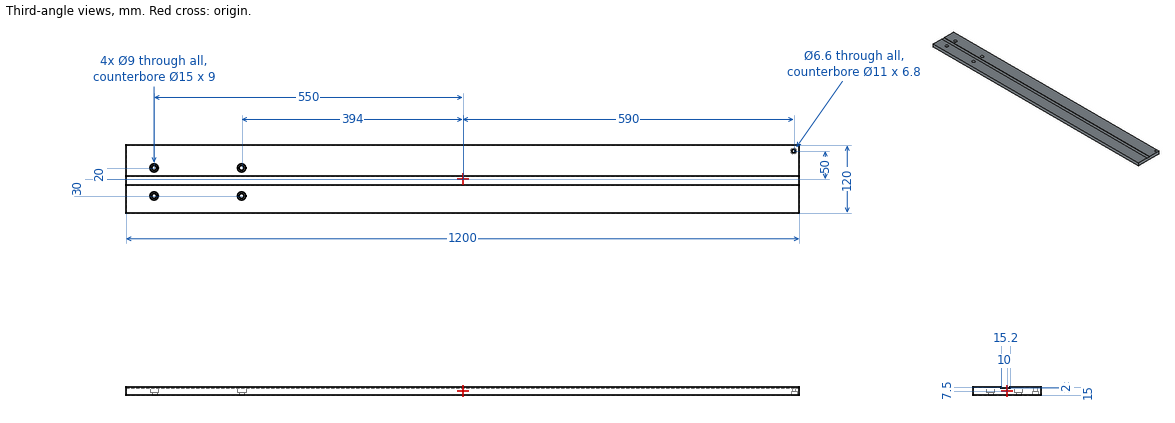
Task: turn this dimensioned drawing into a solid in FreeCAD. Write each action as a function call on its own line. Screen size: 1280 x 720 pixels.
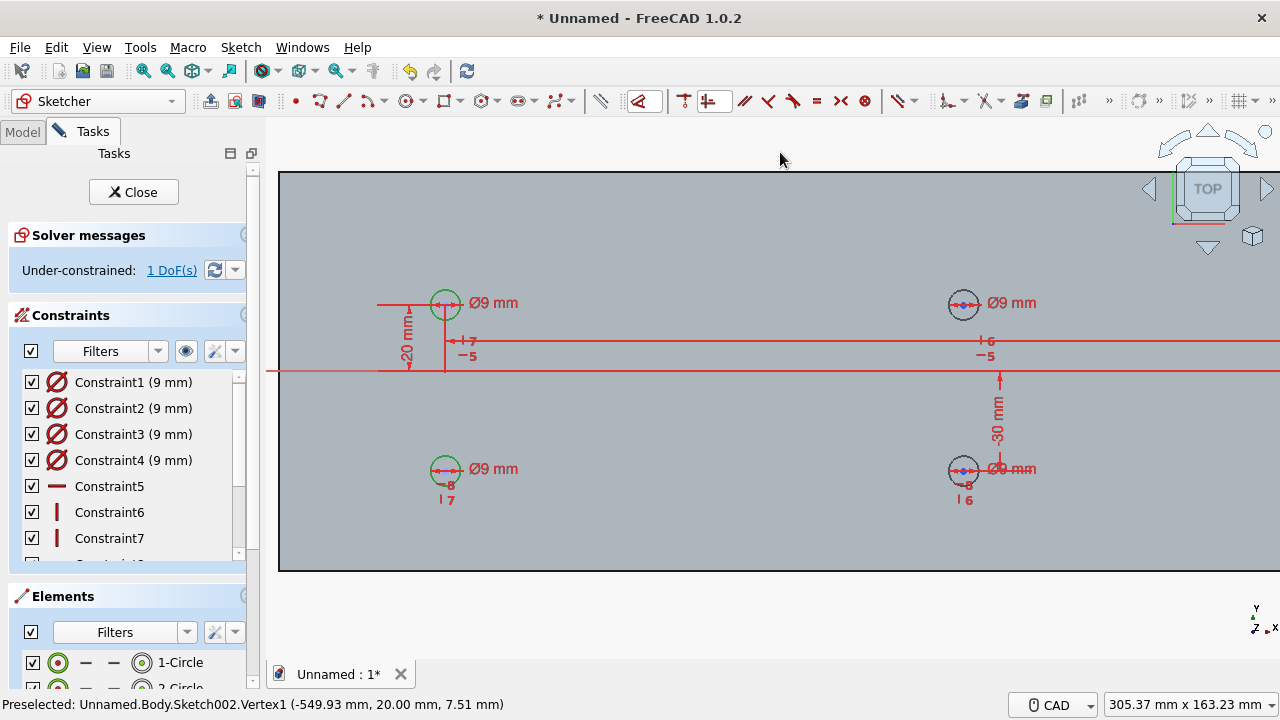
click(964, 305)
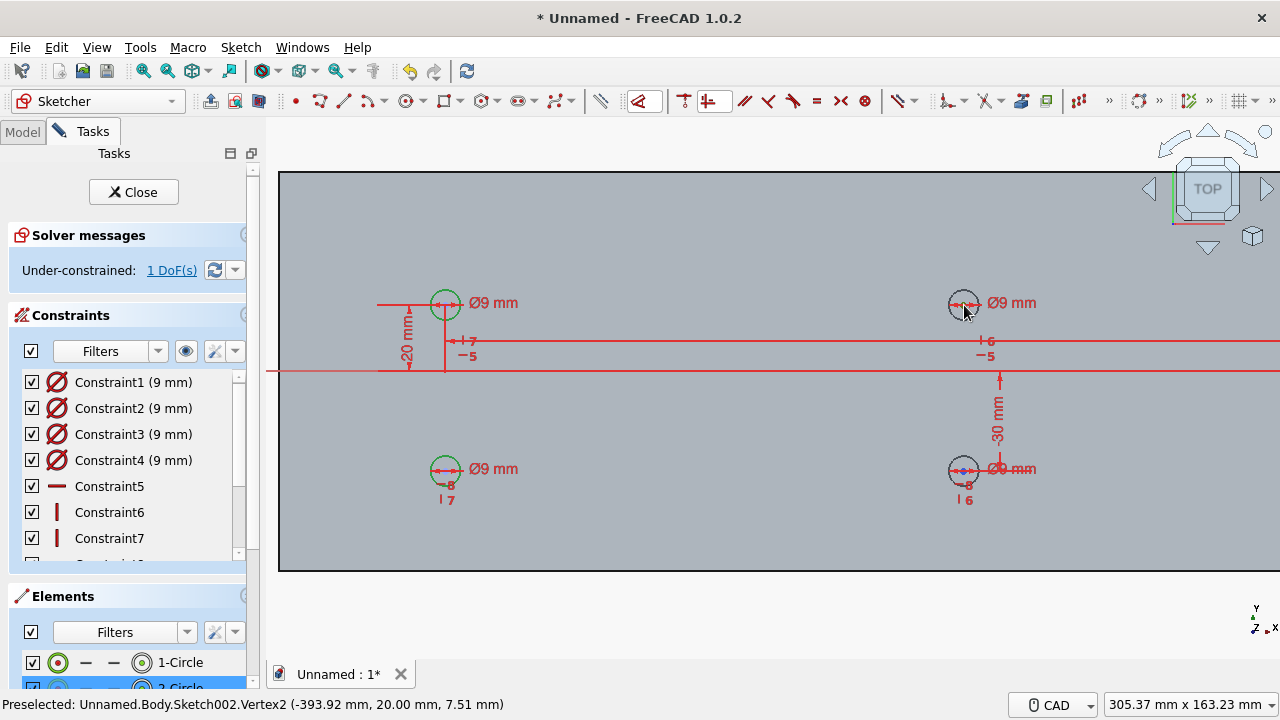
click(656, 102)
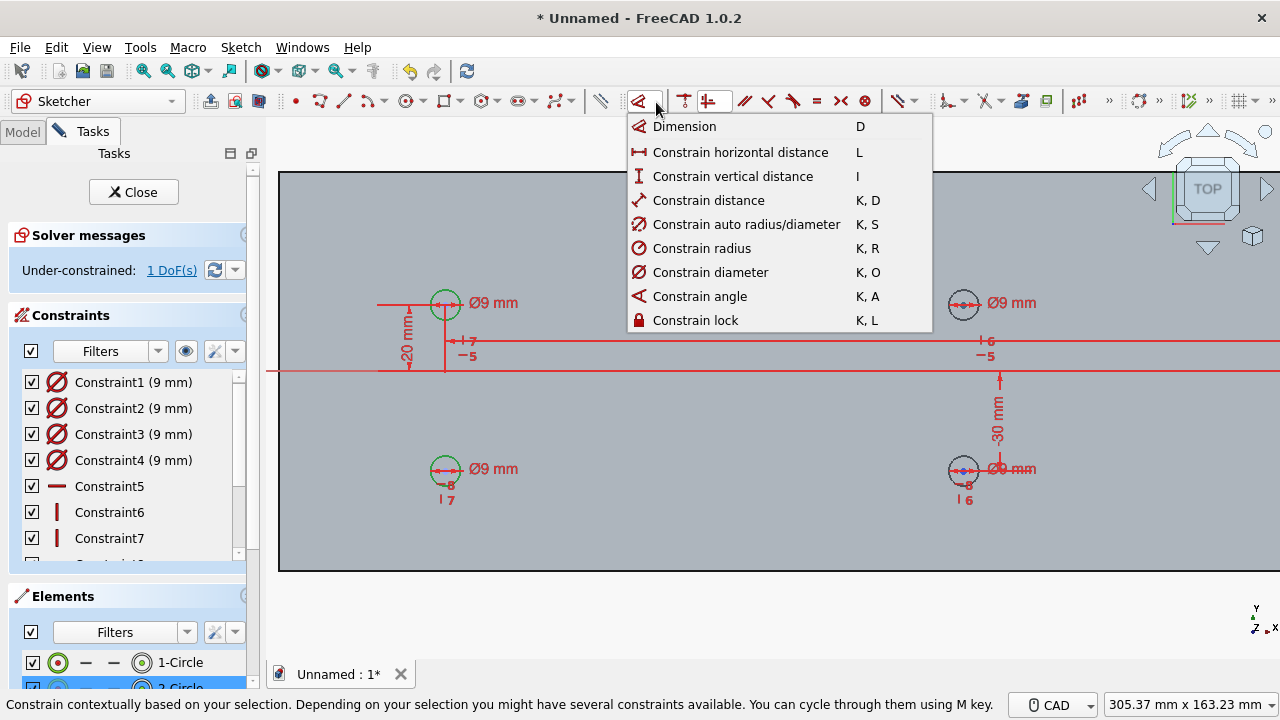
click(780, 152)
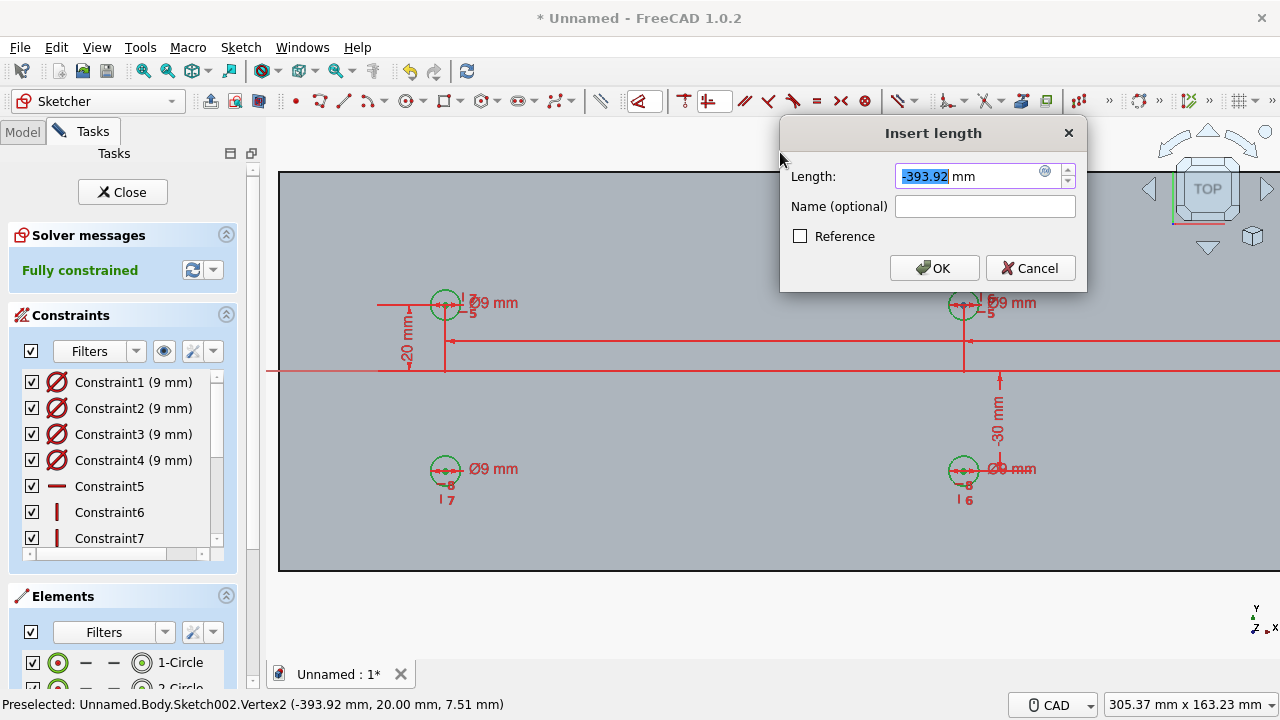
text(-394)
key(Return)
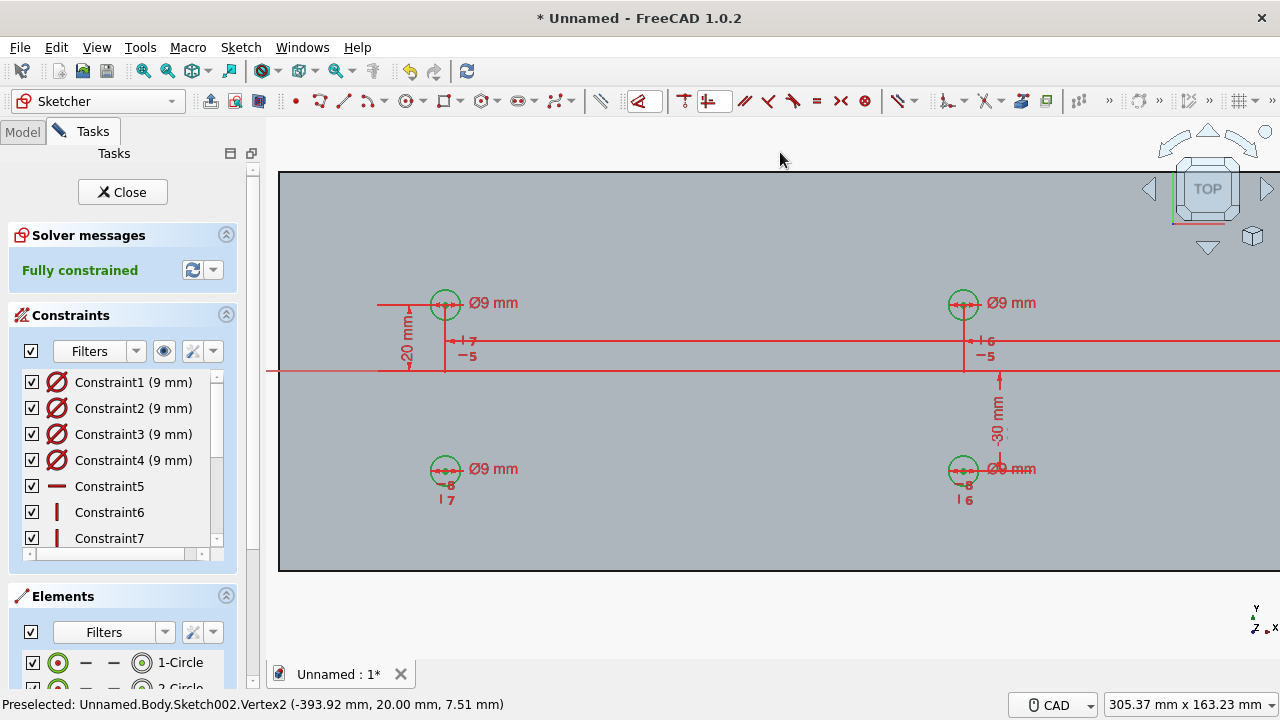
click(123, 192)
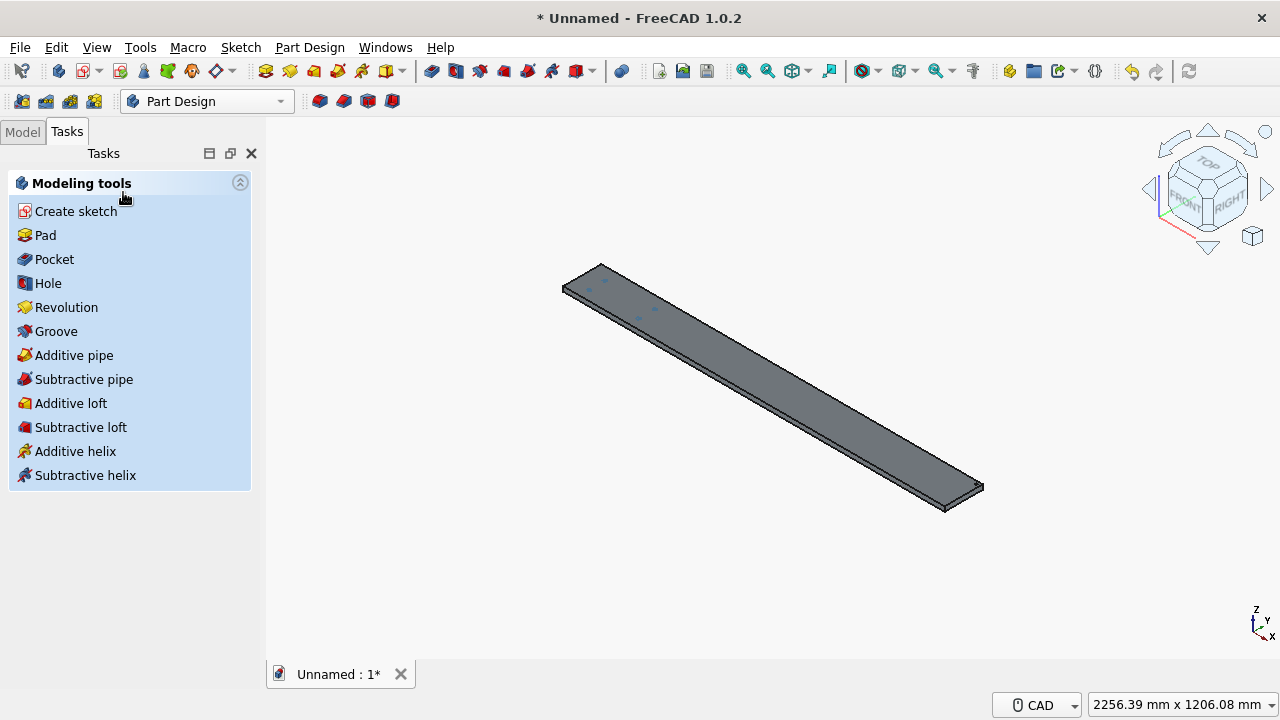
click(456, 72)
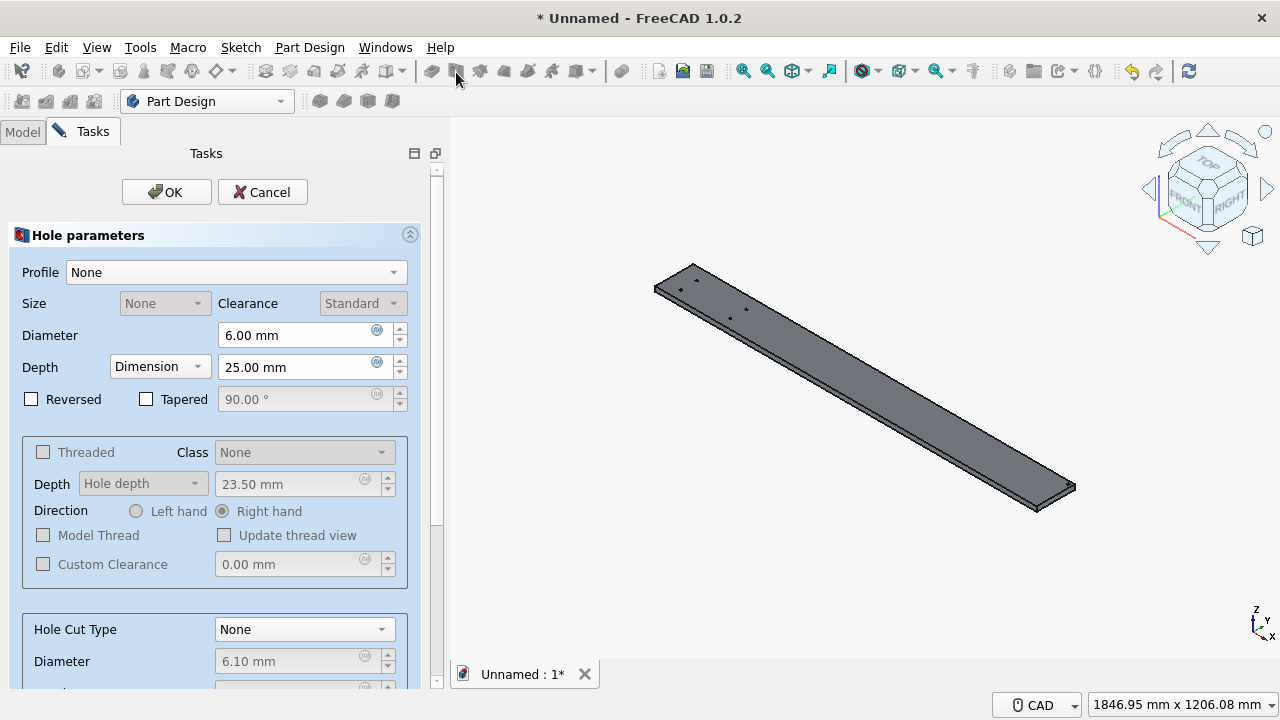
triple_click(305, 335)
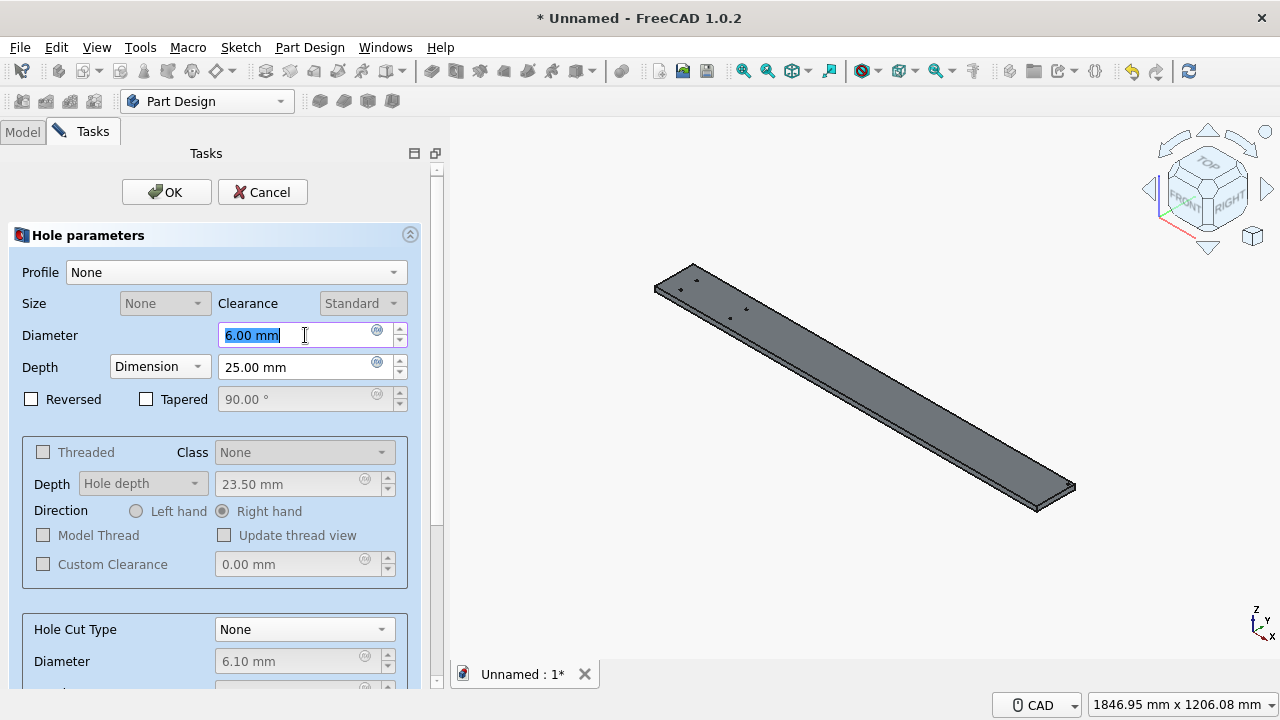
text(9)
key(Tab)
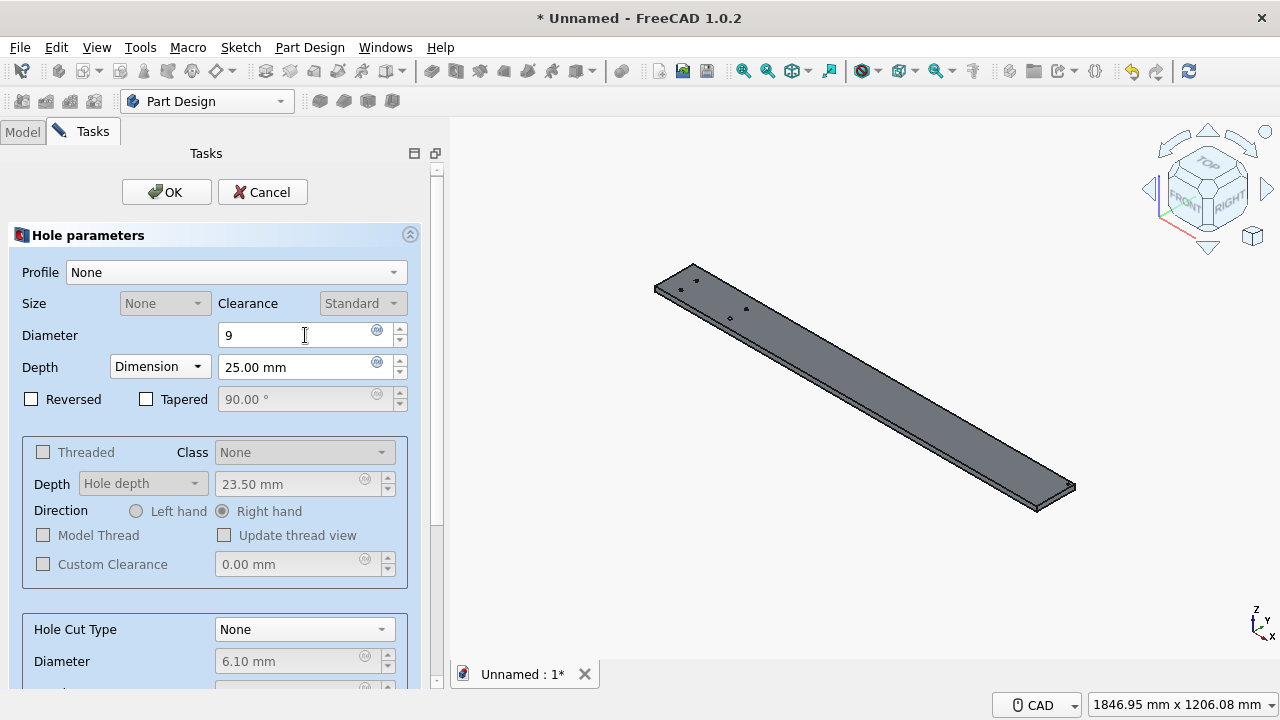
click(161, 366)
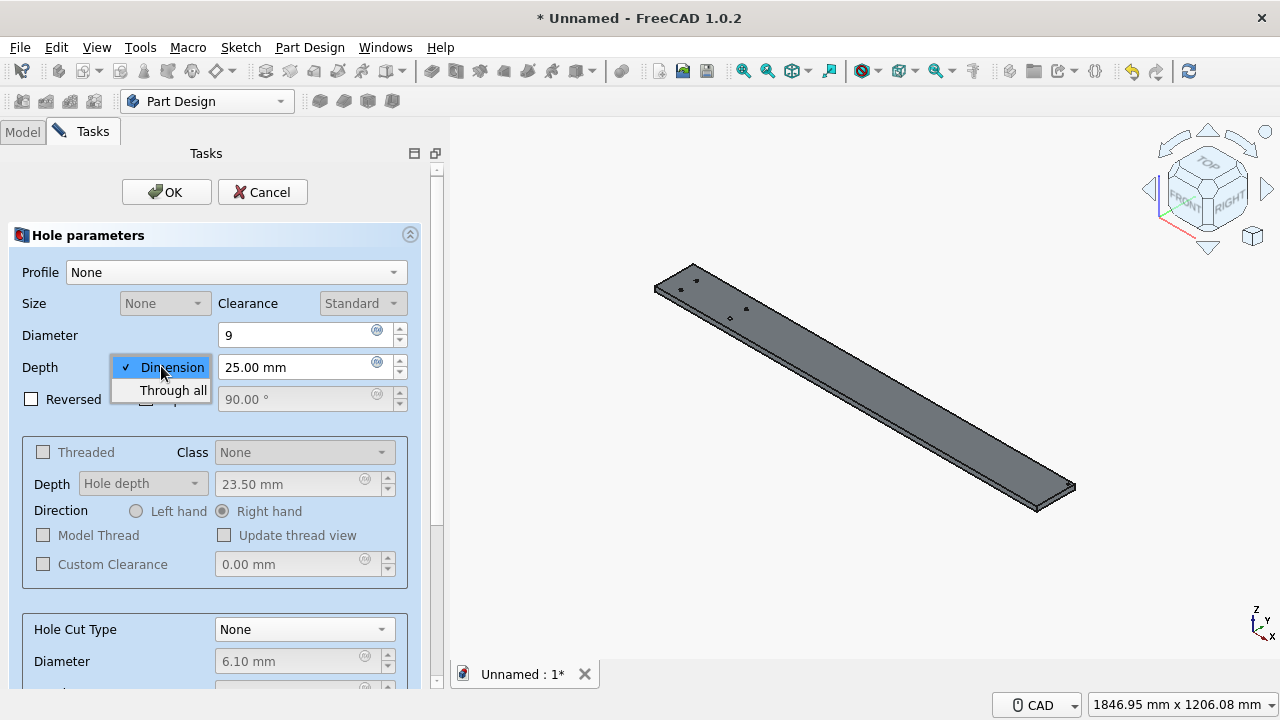
click(160, 390)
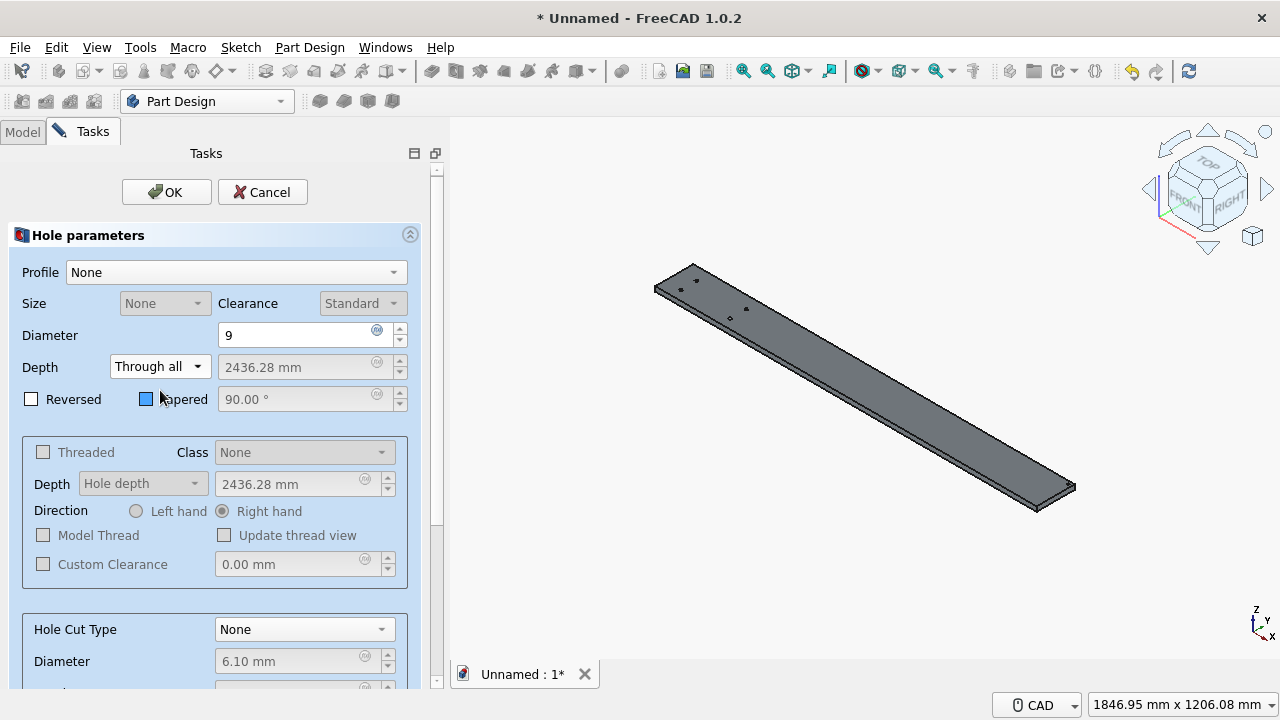
click(306, 630)